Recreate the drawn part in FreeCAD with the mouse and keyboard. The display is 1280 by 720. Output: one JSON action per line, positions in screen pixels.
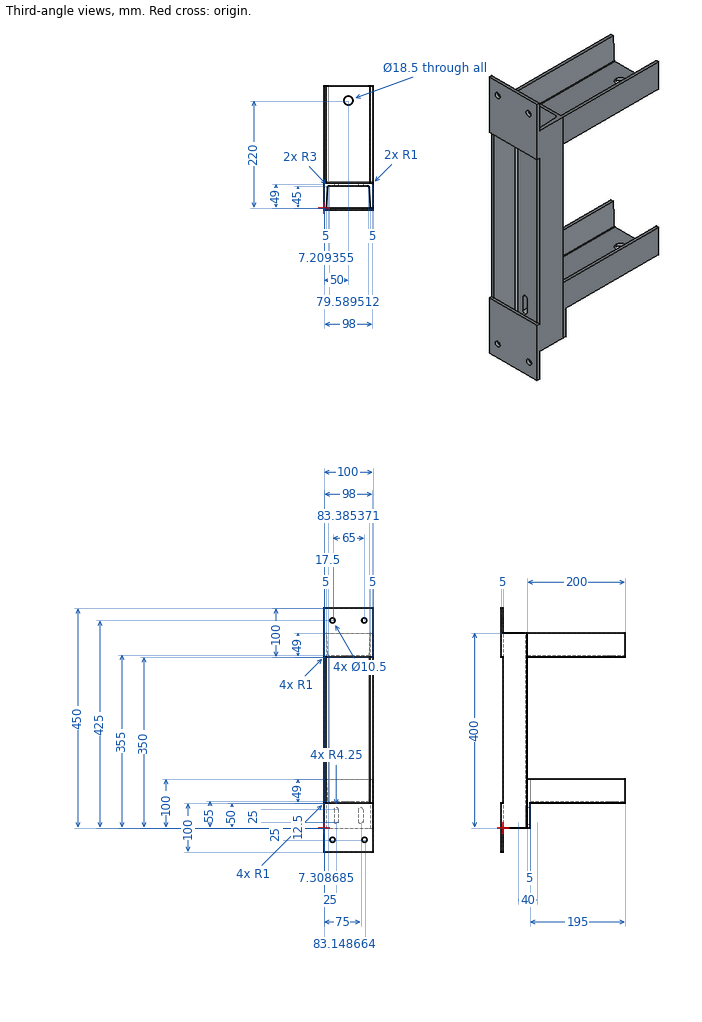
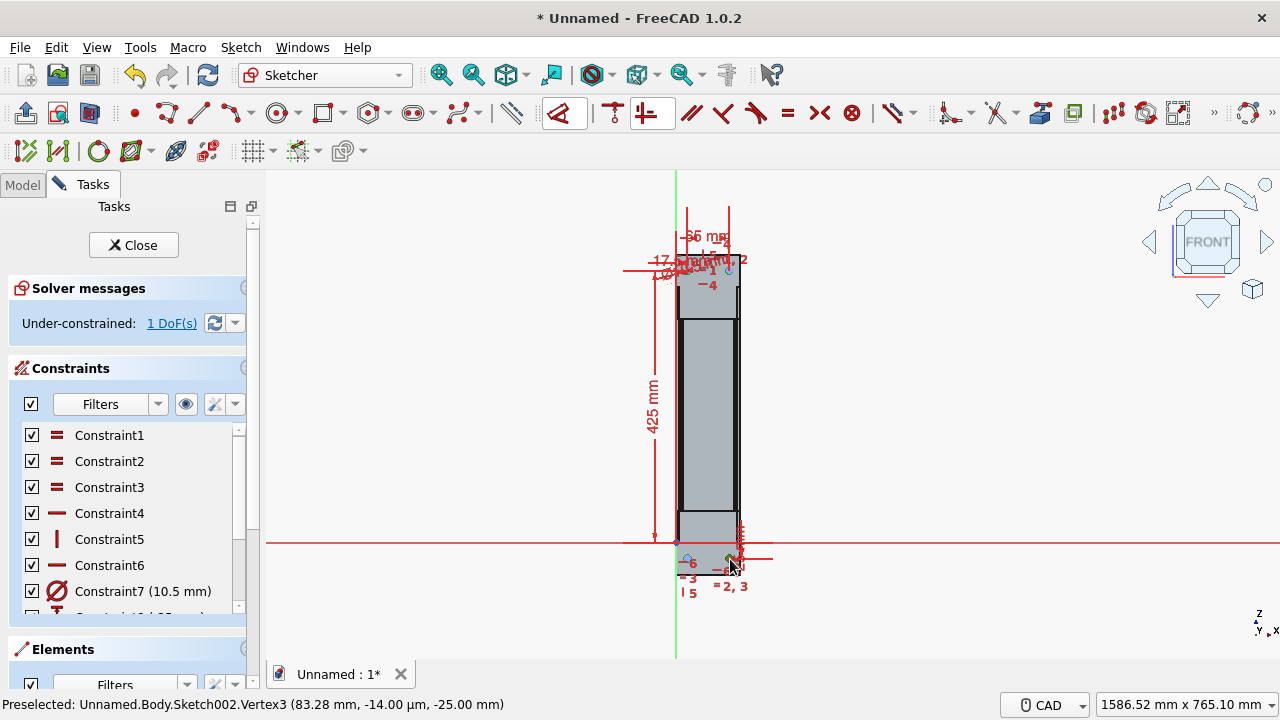
{"action": "key", "text": "l"}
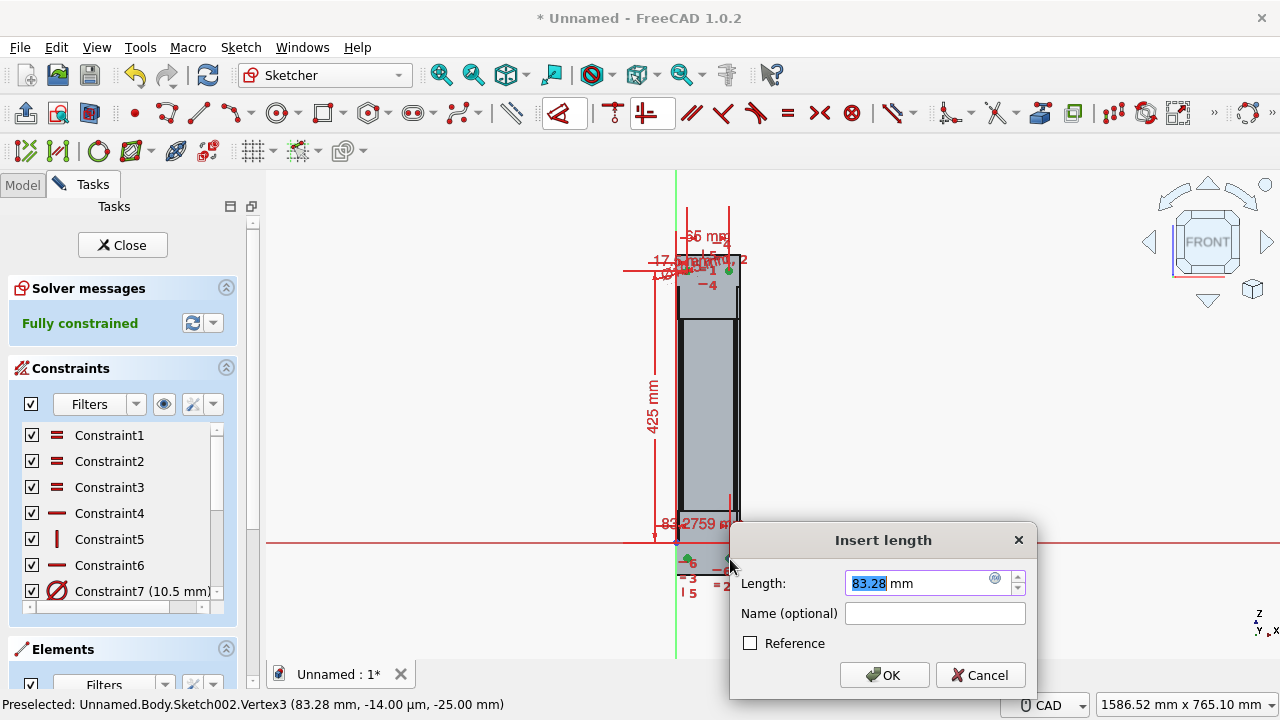
{"action": "type", "text": "83.148664"}
{"action": "key", "text": "Return"}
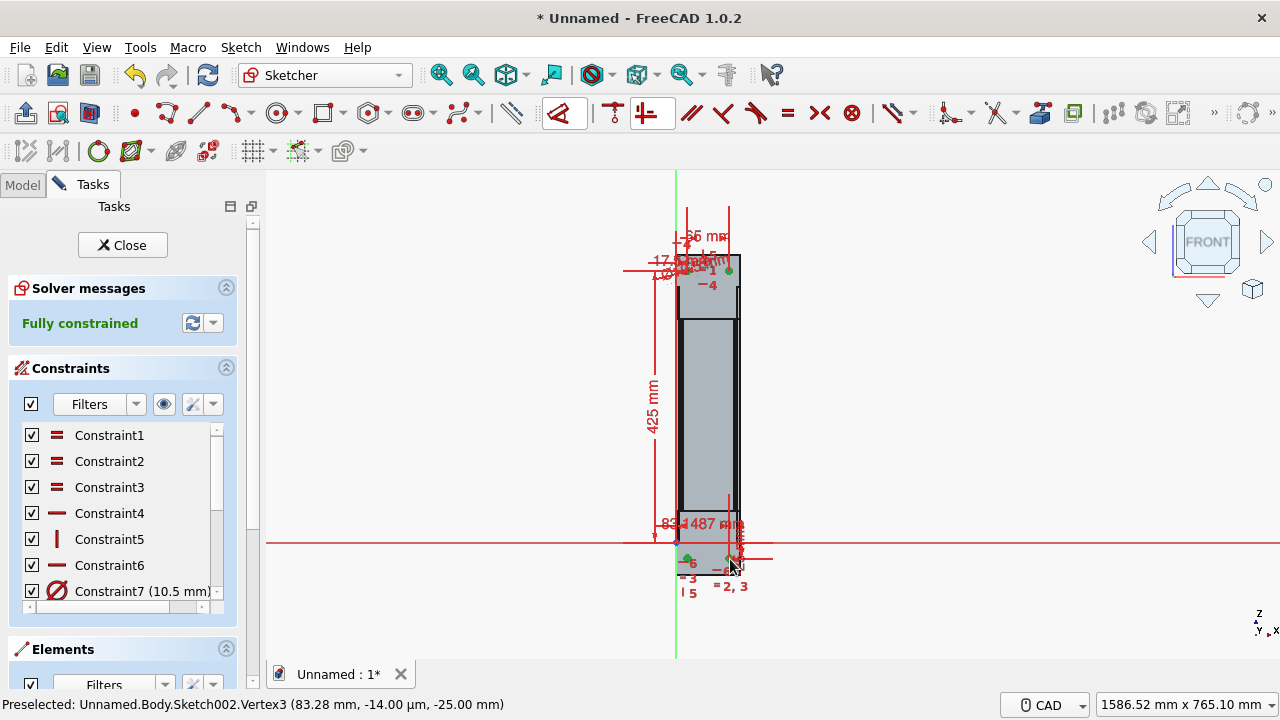
{"action": "left_click", "coordinate": [123, 245]}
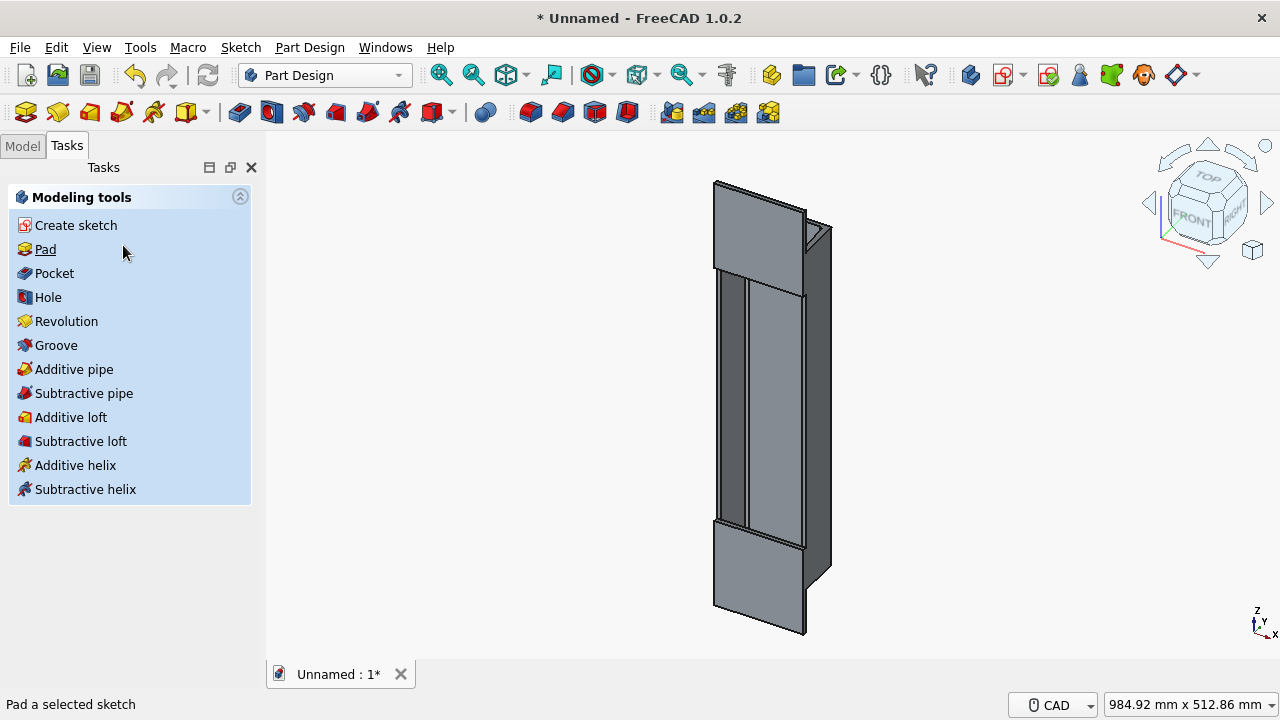
{"action": "left_click", "coordinate": [240, 112]}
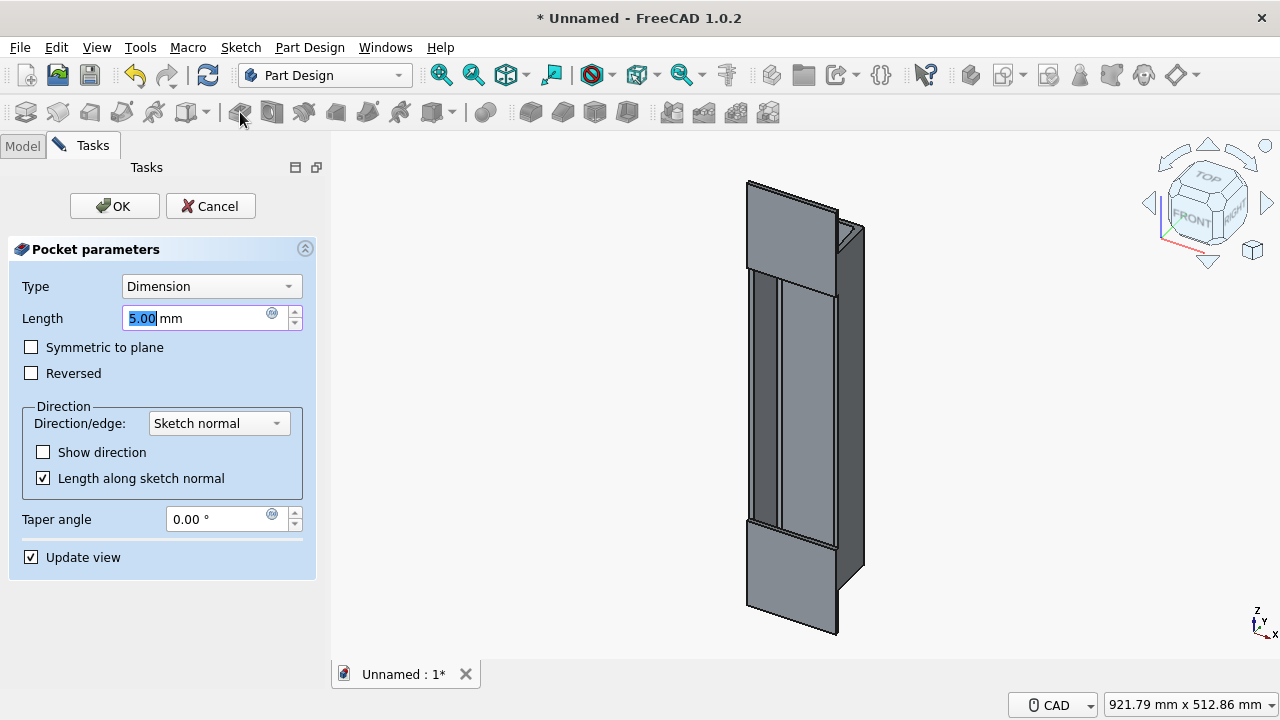
{"action": "left_click", "coordinate": [212, 286]}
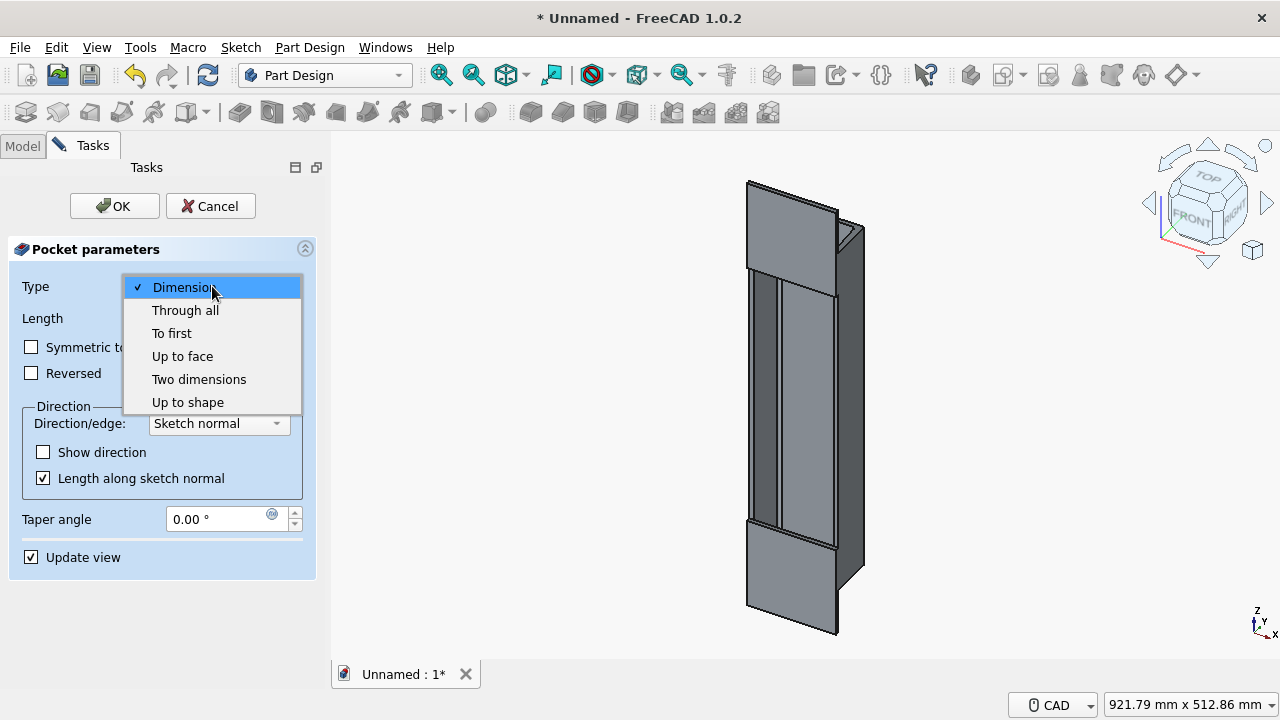
{"action": "left_click", "coordinate": [212, 310]}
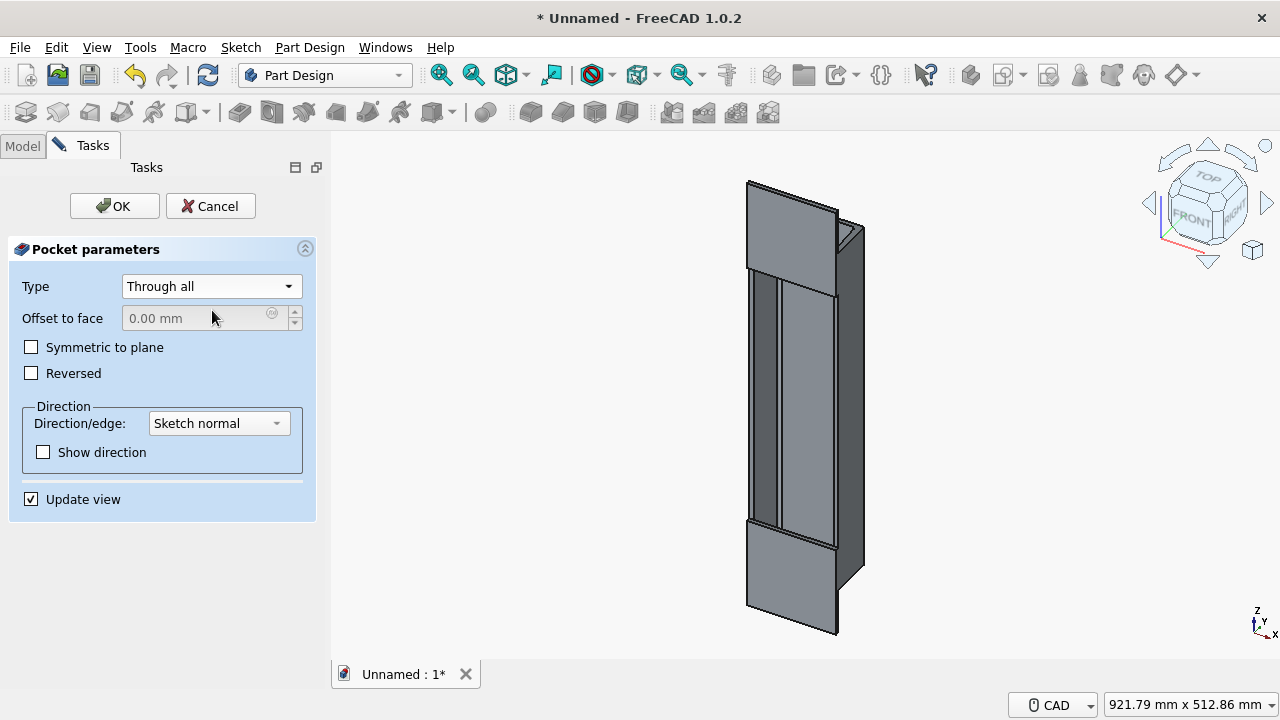
{"action": "left_click", "coordinate": [30, 373]}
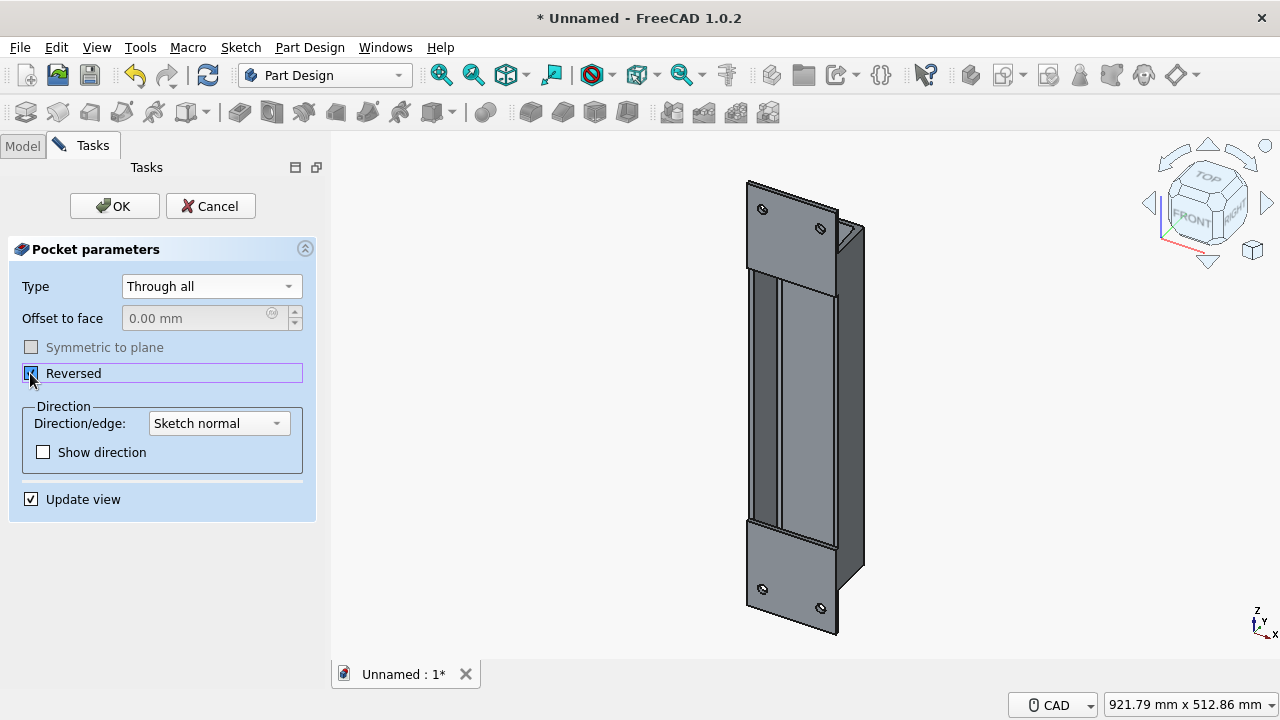
{"action": "left_click", "coordinate": [115, 206]}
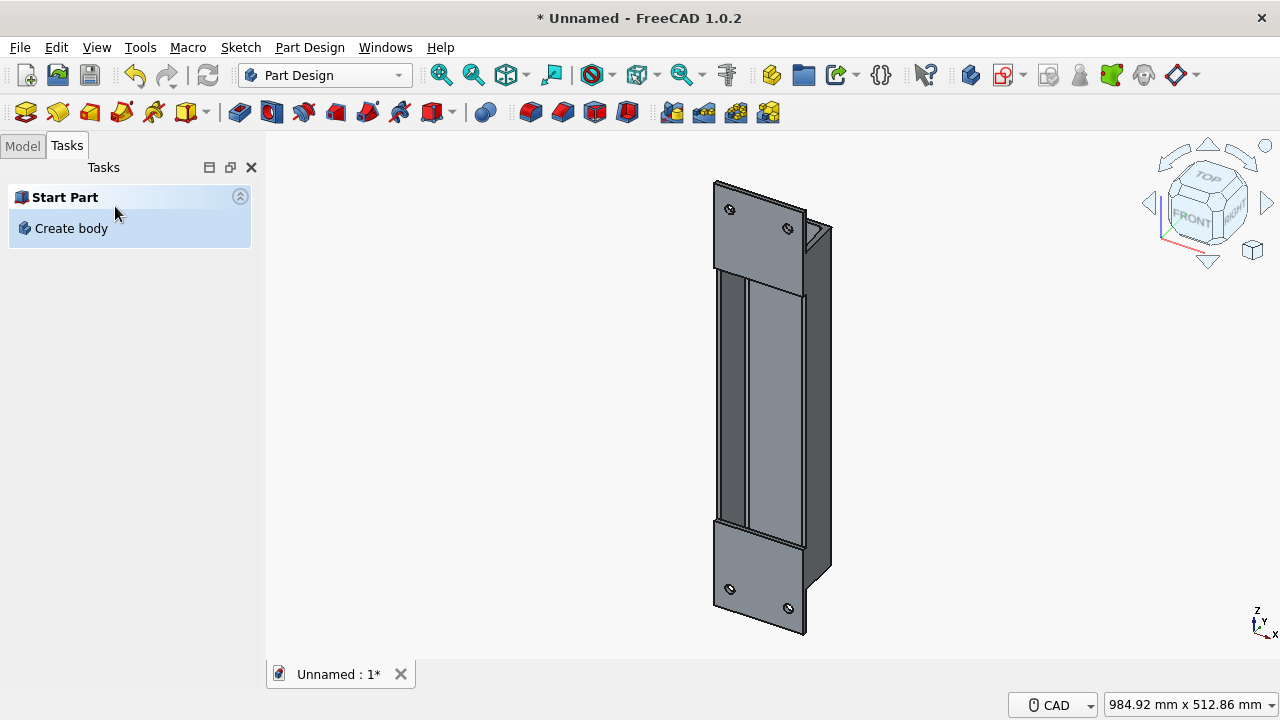
{"action": "key", "text": "4"}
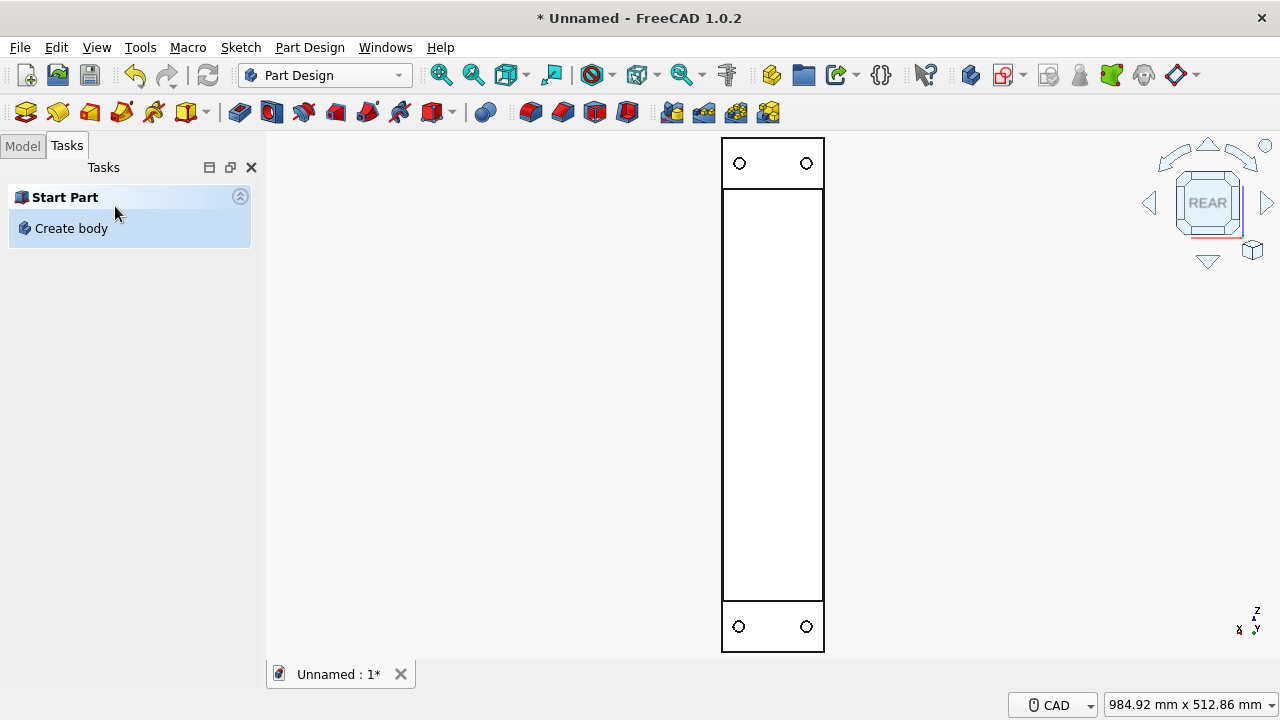
{"action": "left_click", "coordinate": [773, 276]}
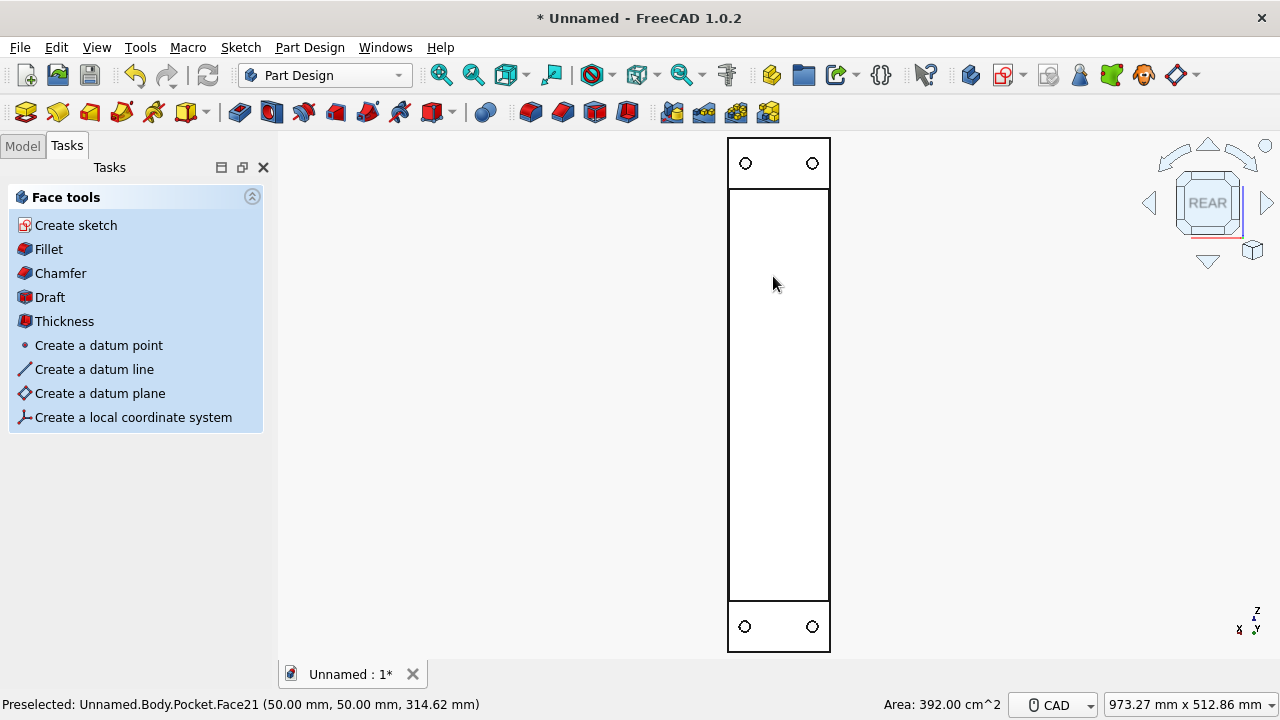
{"action": "left_click", "coordinate": [1004, 76]}